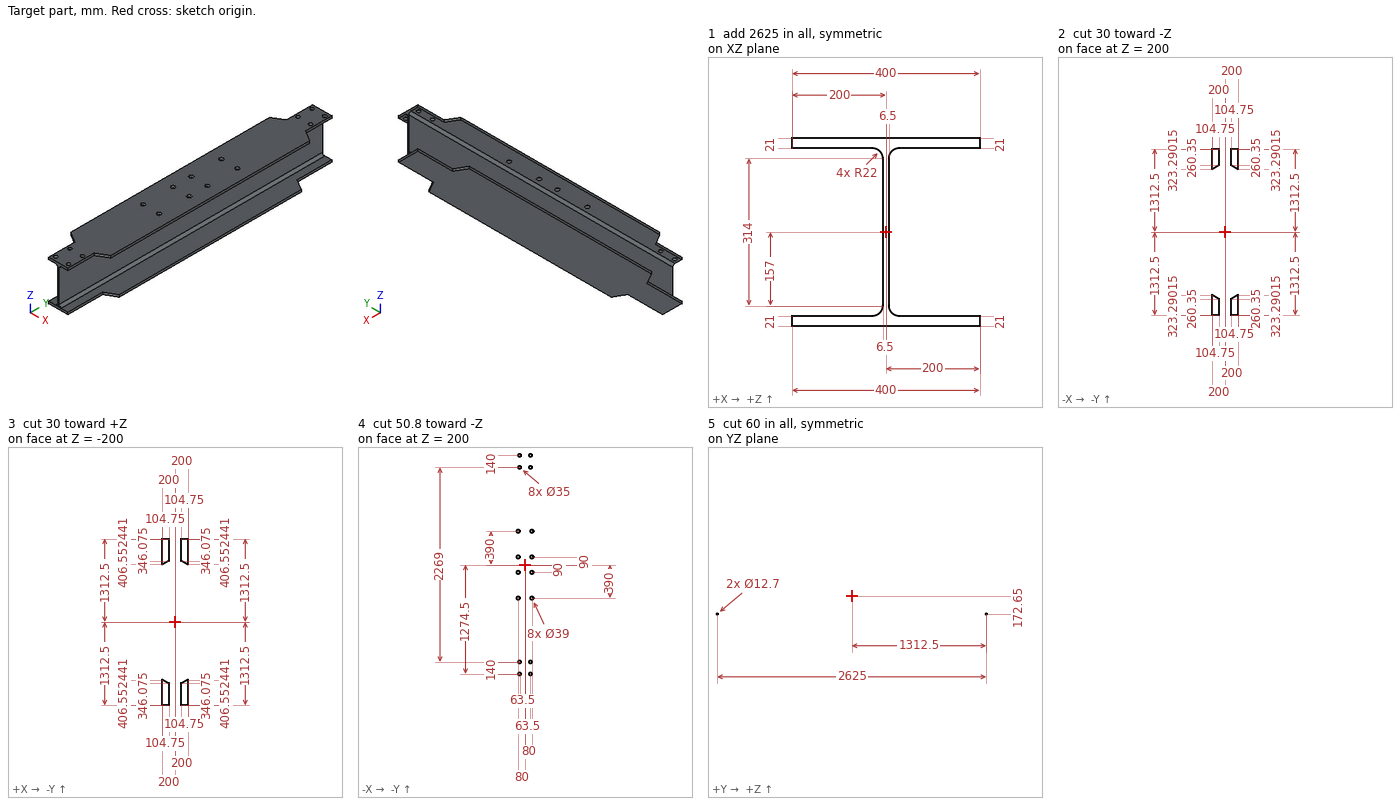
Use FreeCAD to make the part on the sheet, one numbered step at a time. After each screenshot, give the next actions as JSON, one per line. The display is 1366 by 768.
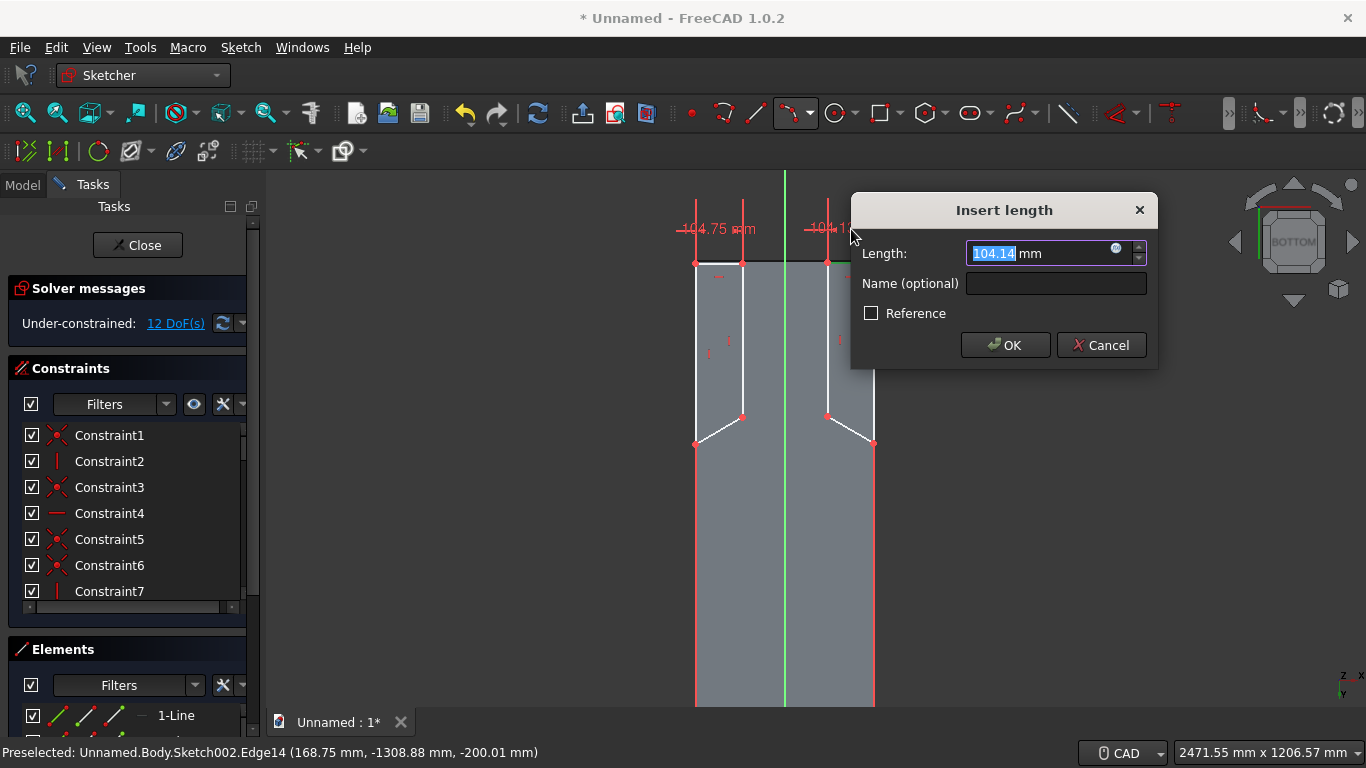
{"action": "type", "text": "104.75"}
{"action": "key", "text": "Return"}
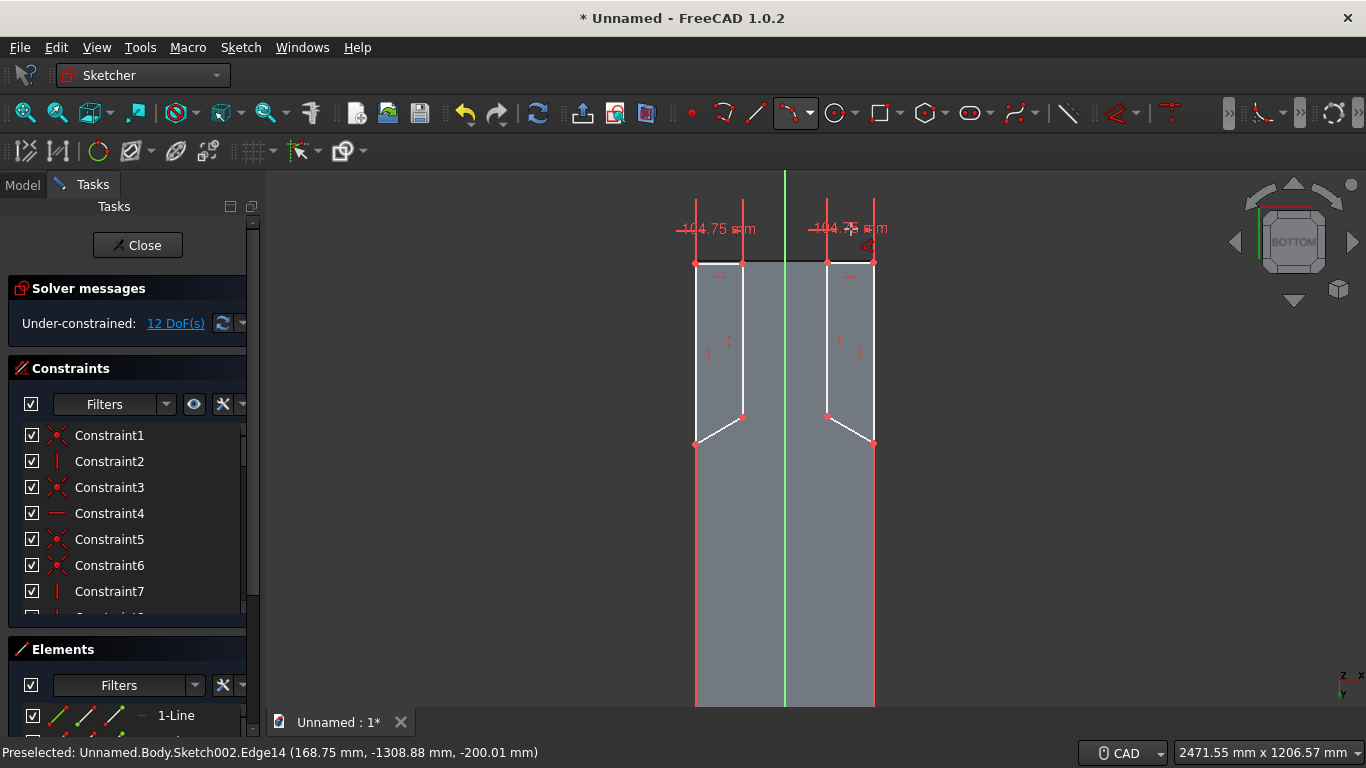
{"action": "scroll", "coordinate": [731, 263], "scroll_direction": "down", "scroll_amount": 6}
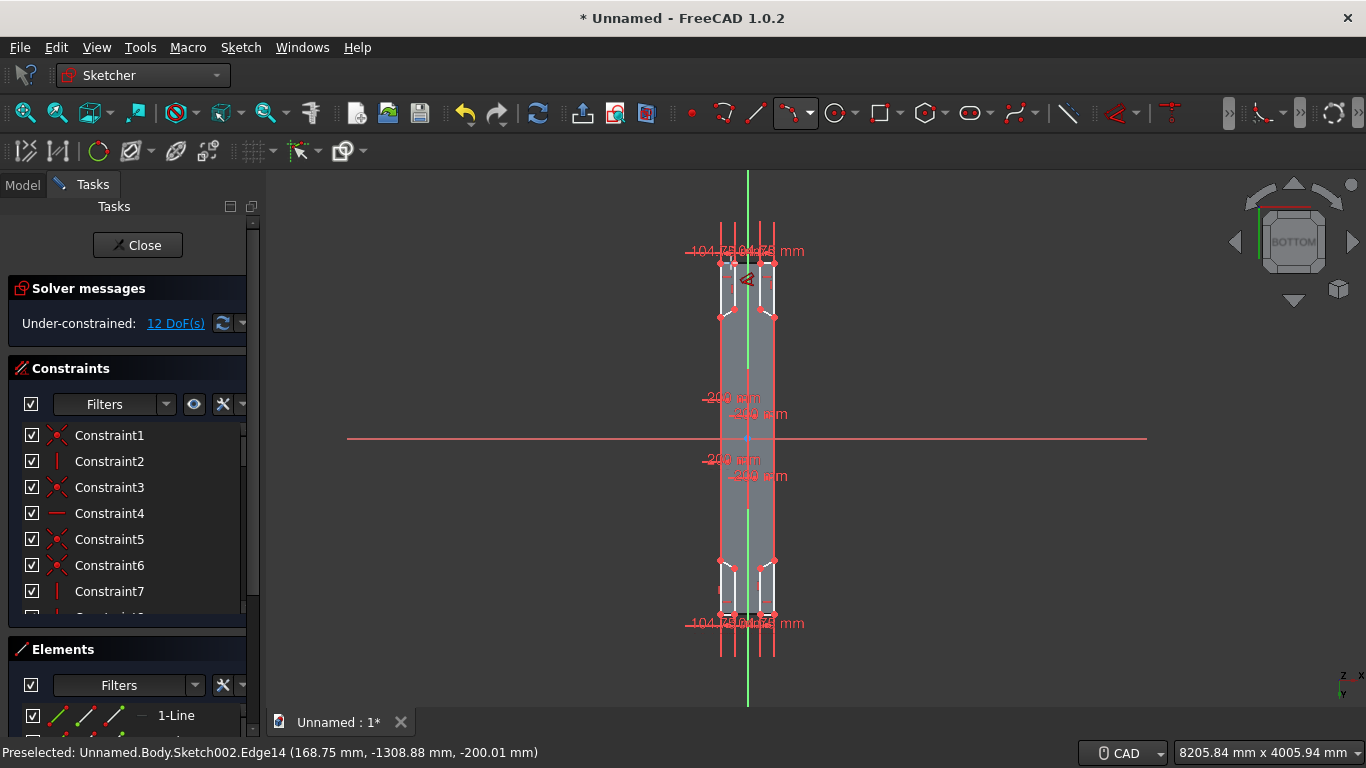
{"action": "left_click", "coordinate": [760, 582]}
{"action": "left_click", "coordinate": [794, 592]}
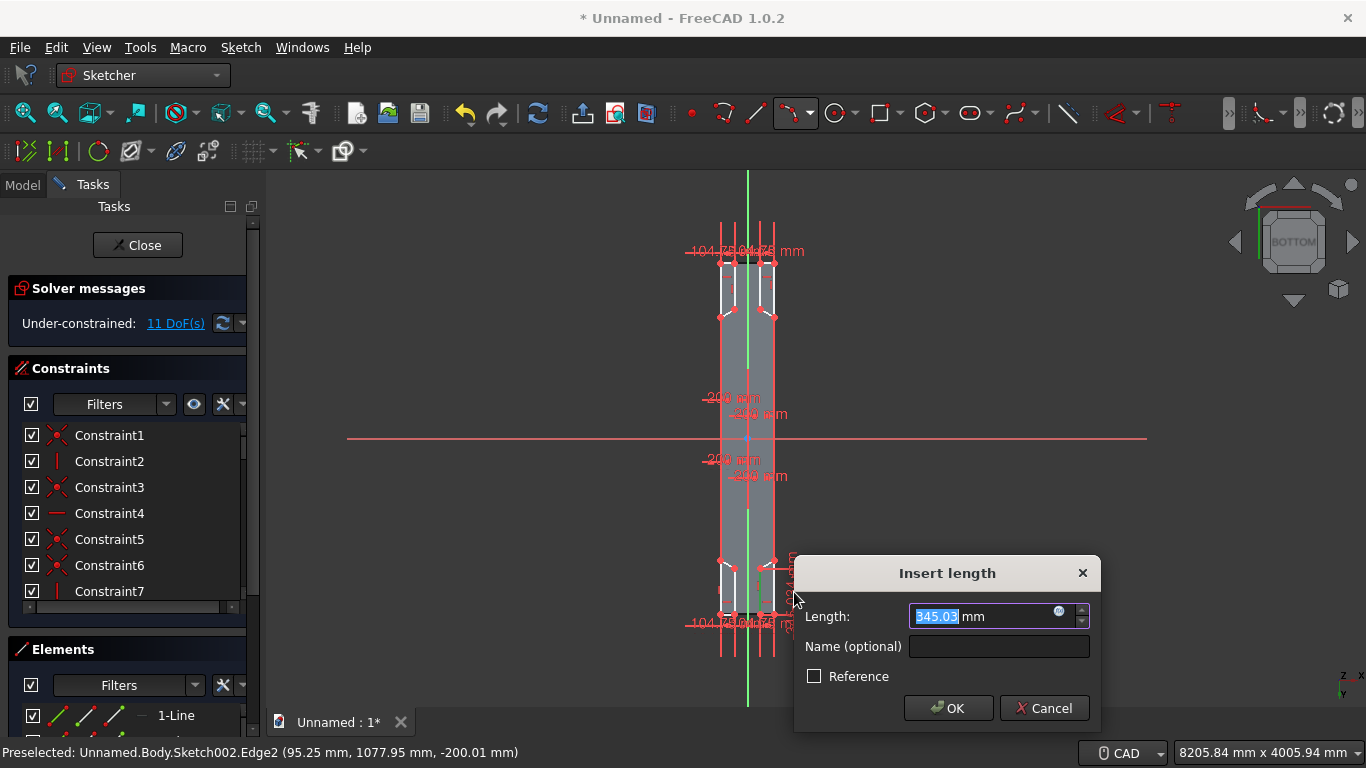
{"action": "type", "text": "346.075"}
{"action": "key", "text": "Return"}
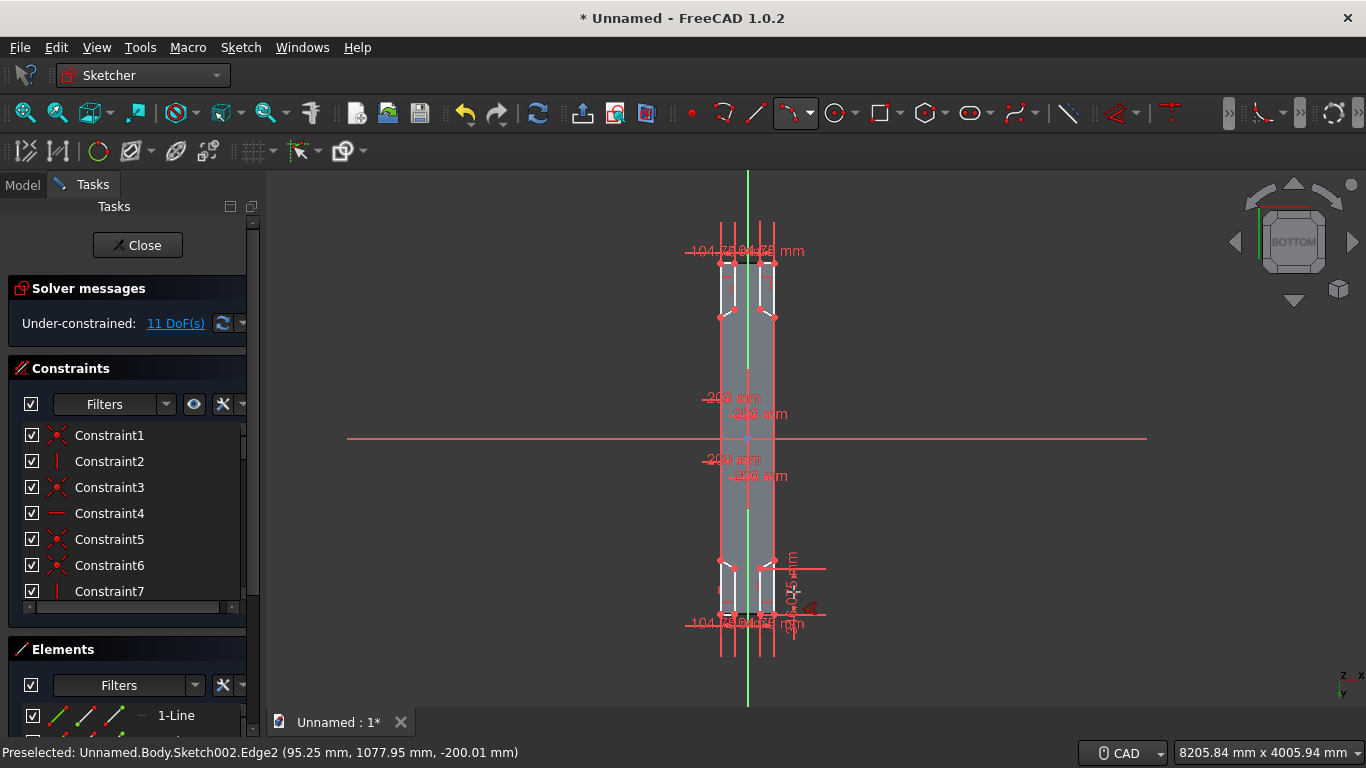
{"action": "left_click", "coordinate": [735, 601]}
{"action": "left_click", "coordinate": [701, 592]}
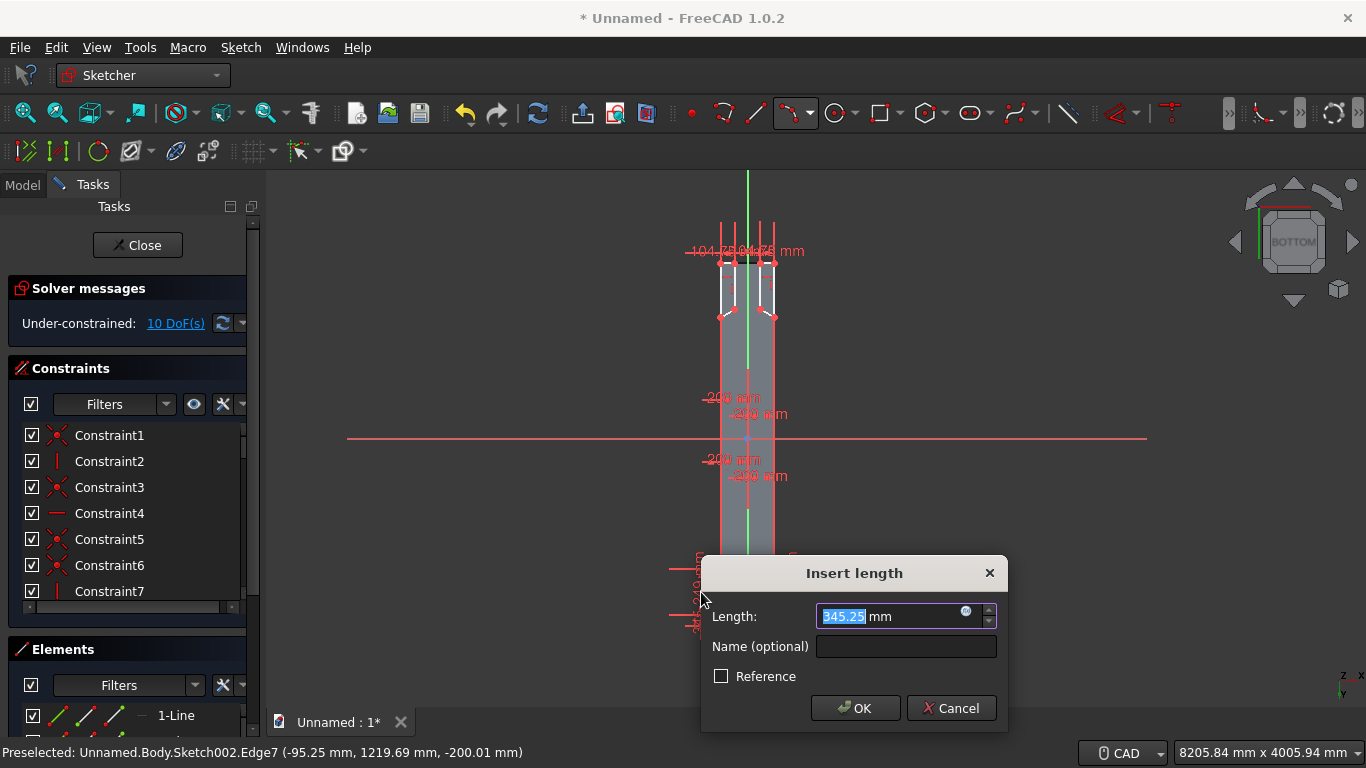
{"action": "type", "text": "346.075"}
{"action": "key", "text": "Return"}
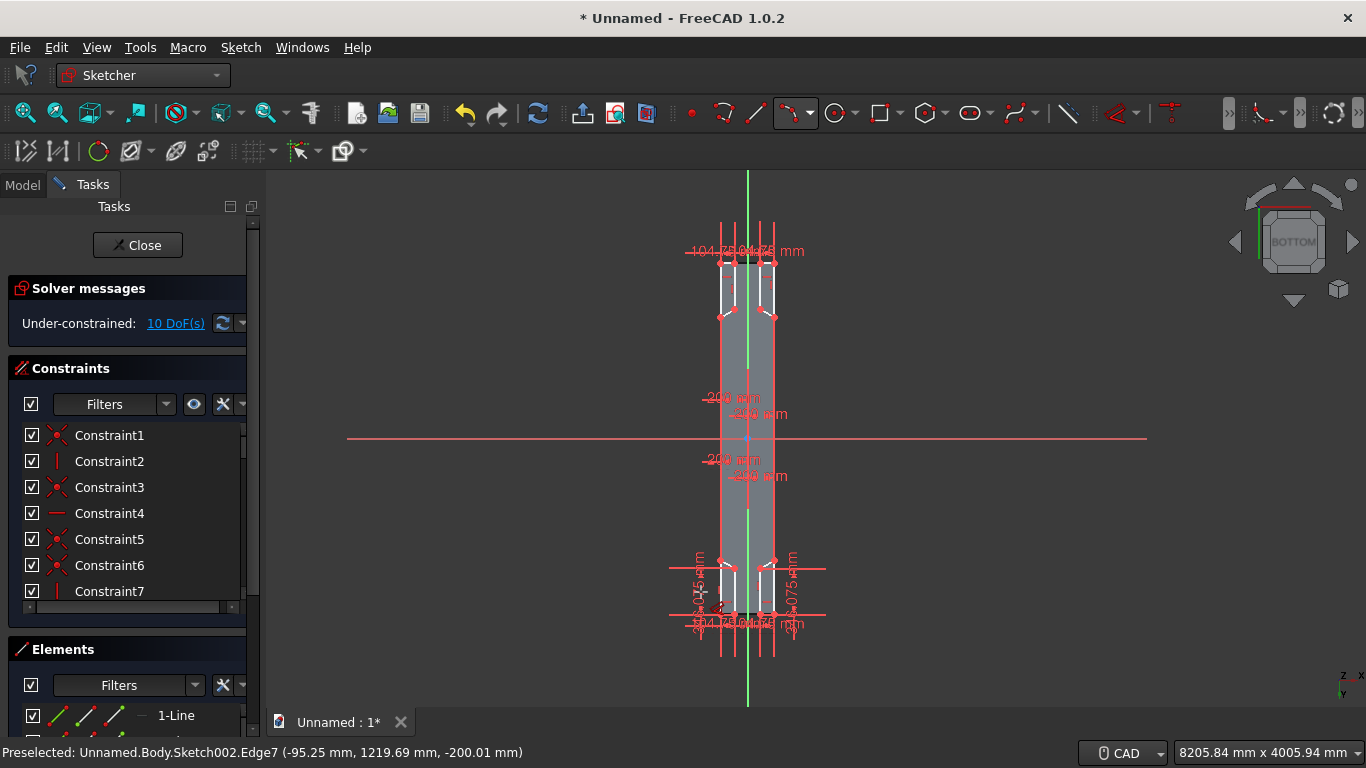
{"action": "left_click", "coordinate": [735, 296]}
{"action": "left_click", "coordinate": [701, 286]}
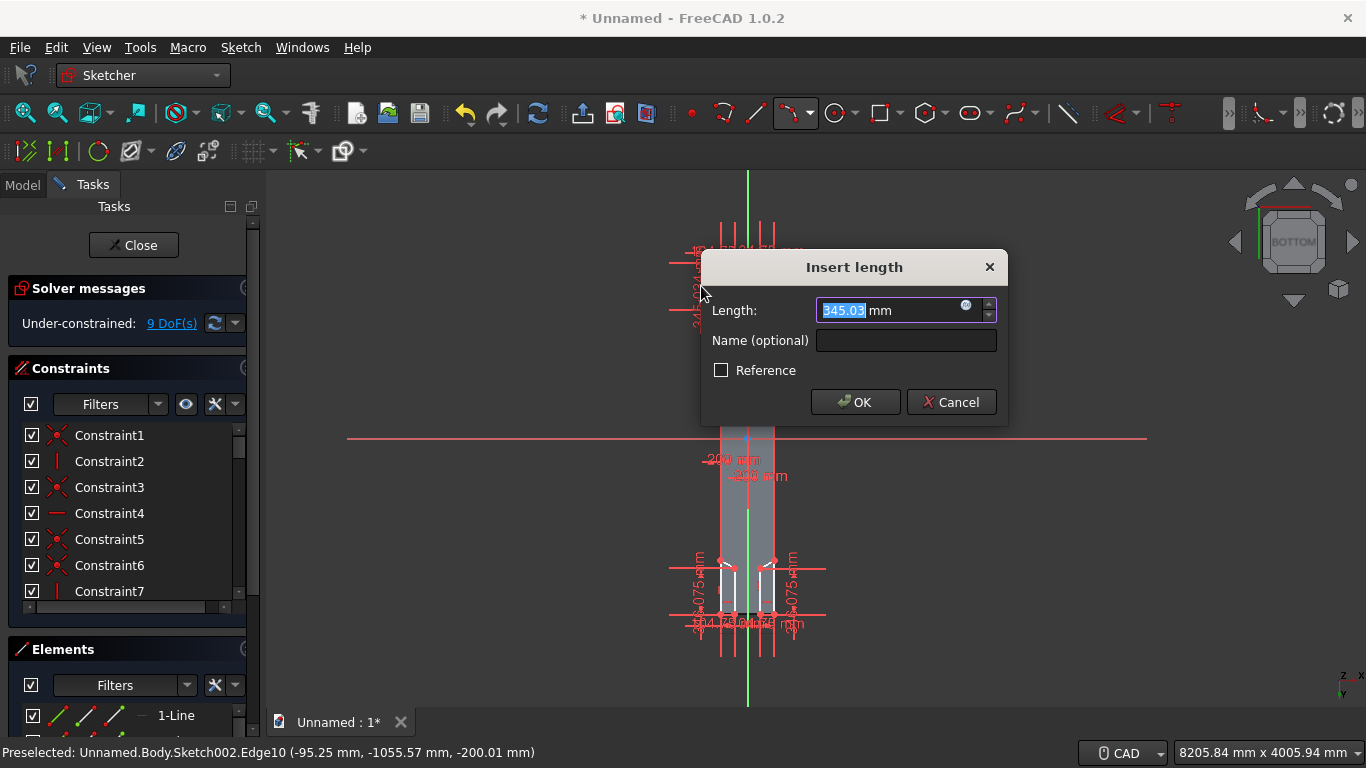
{"action": "type", "text": "346.075"}
{"action": "key", "text": "Return"}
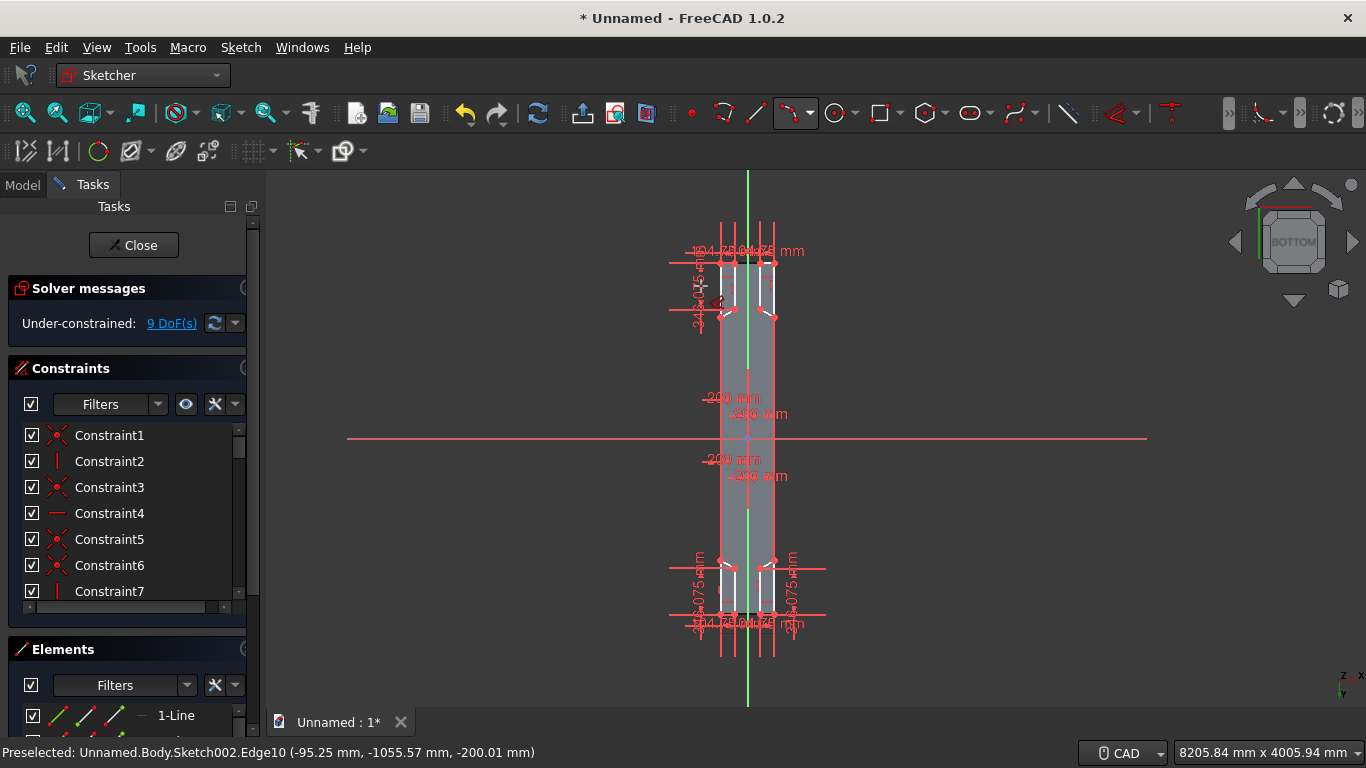
{"action": "left_click", "coordinate": [760, 277]}
{"action": "left_click", "coordinate": [794, 286]}